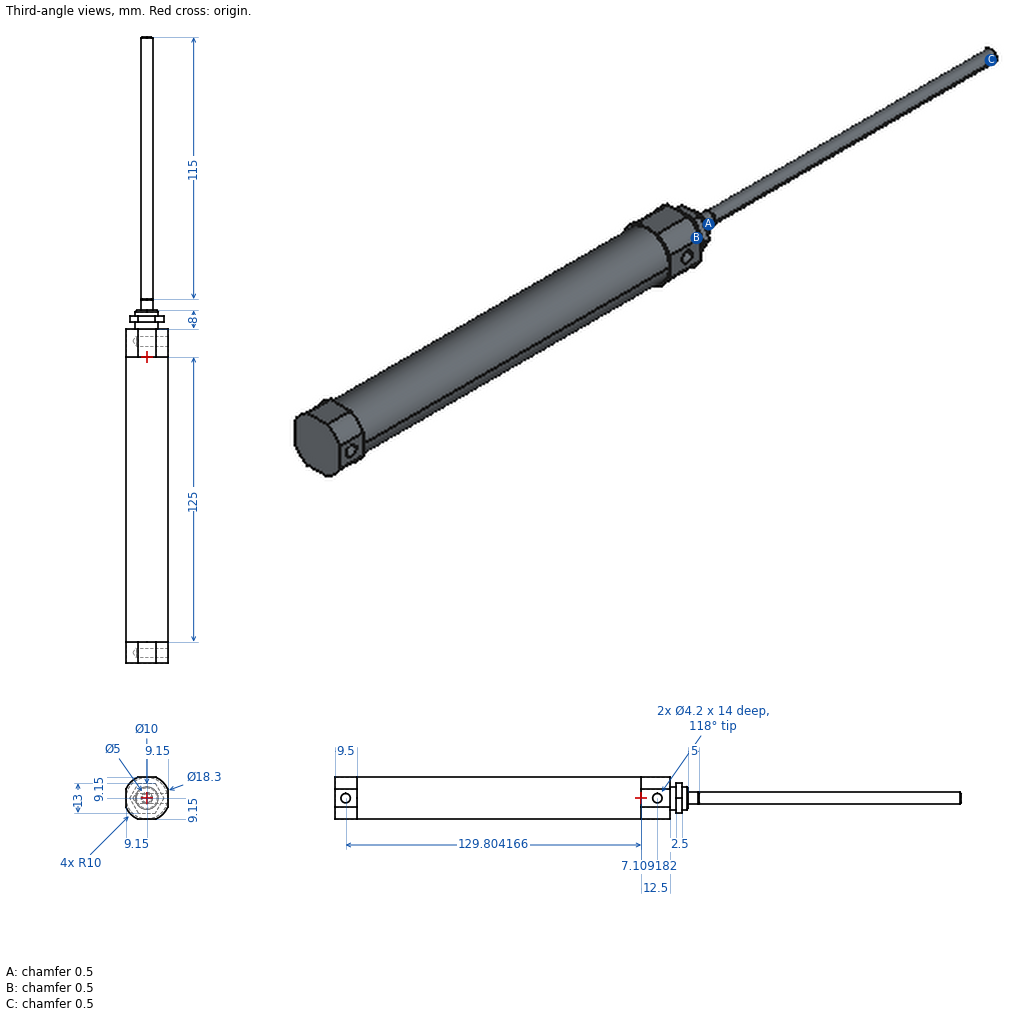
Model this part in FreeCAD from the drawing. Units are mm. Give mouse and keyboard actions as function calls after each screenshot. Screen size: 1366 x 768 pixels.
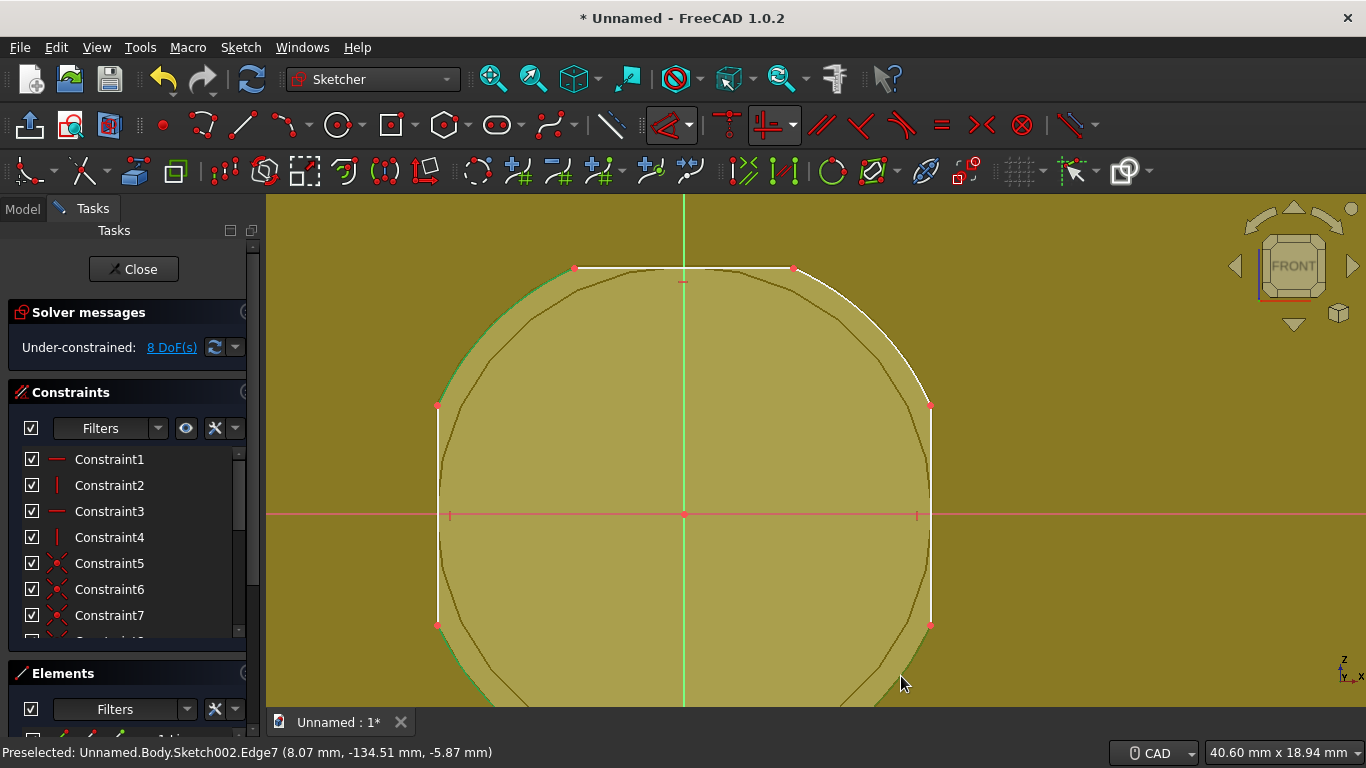
click(901, 354)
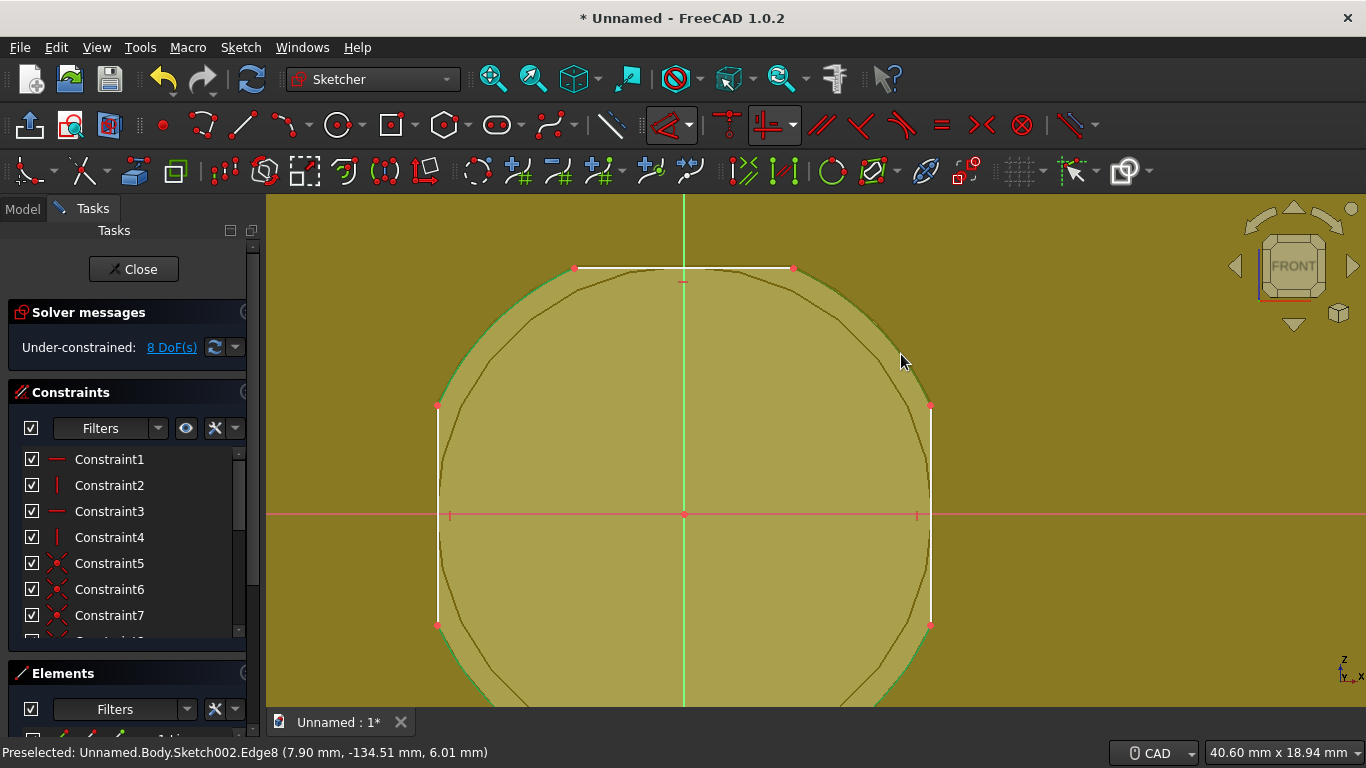
key(e)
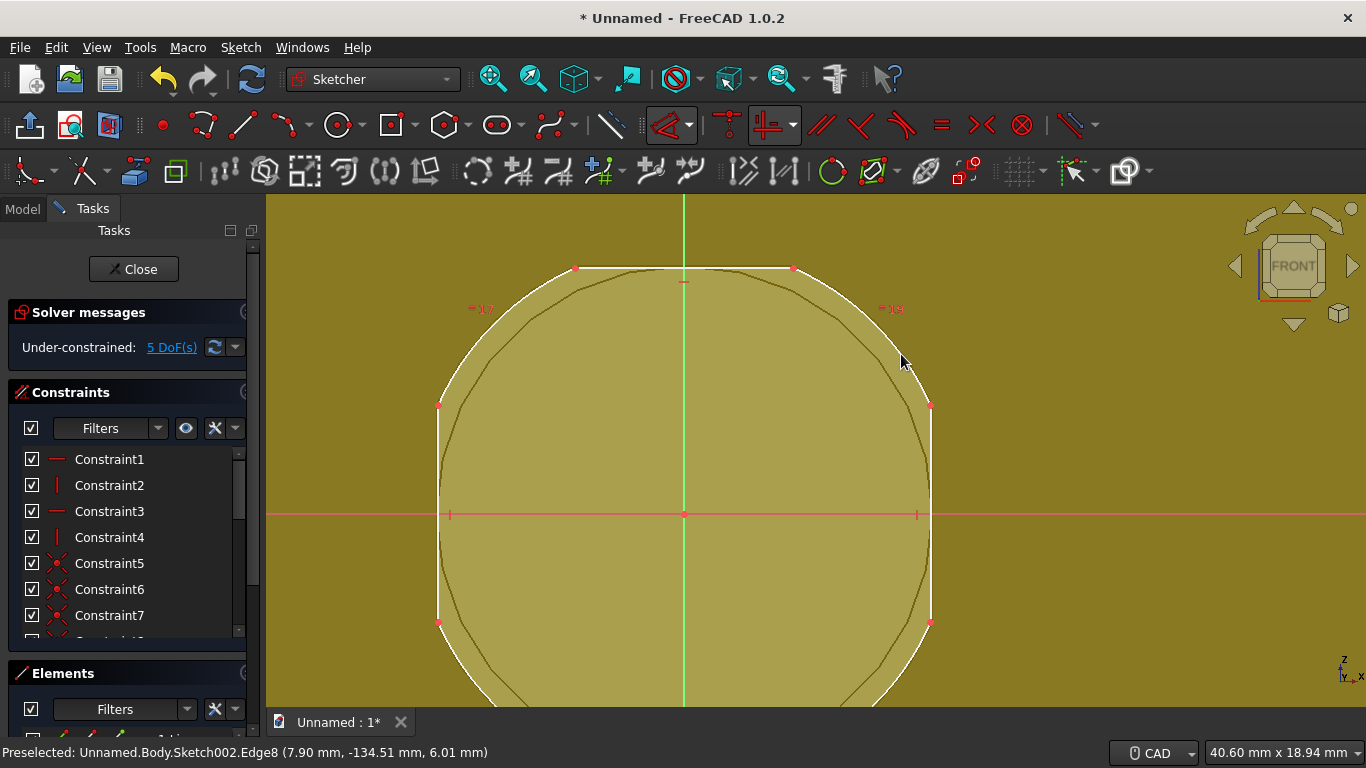
key(d)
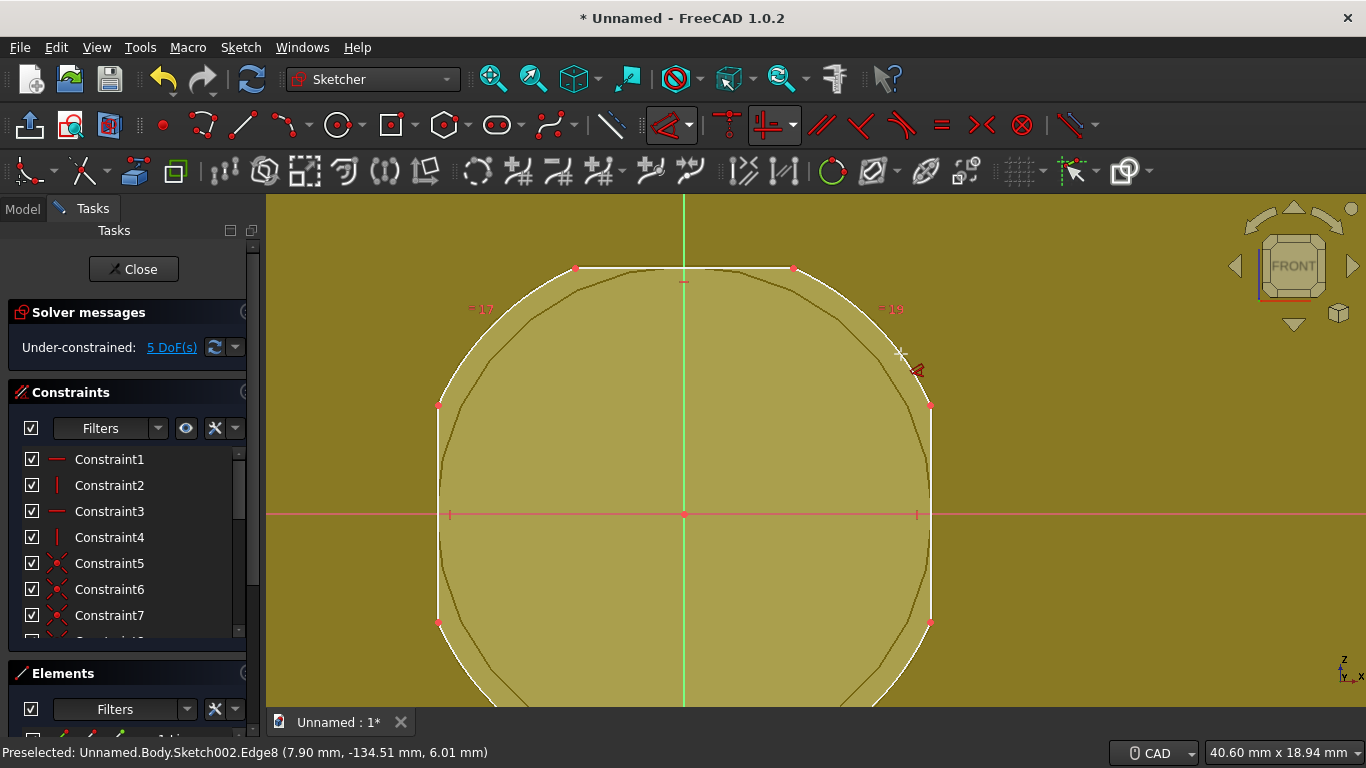
click(524, 298)
click(505, 272)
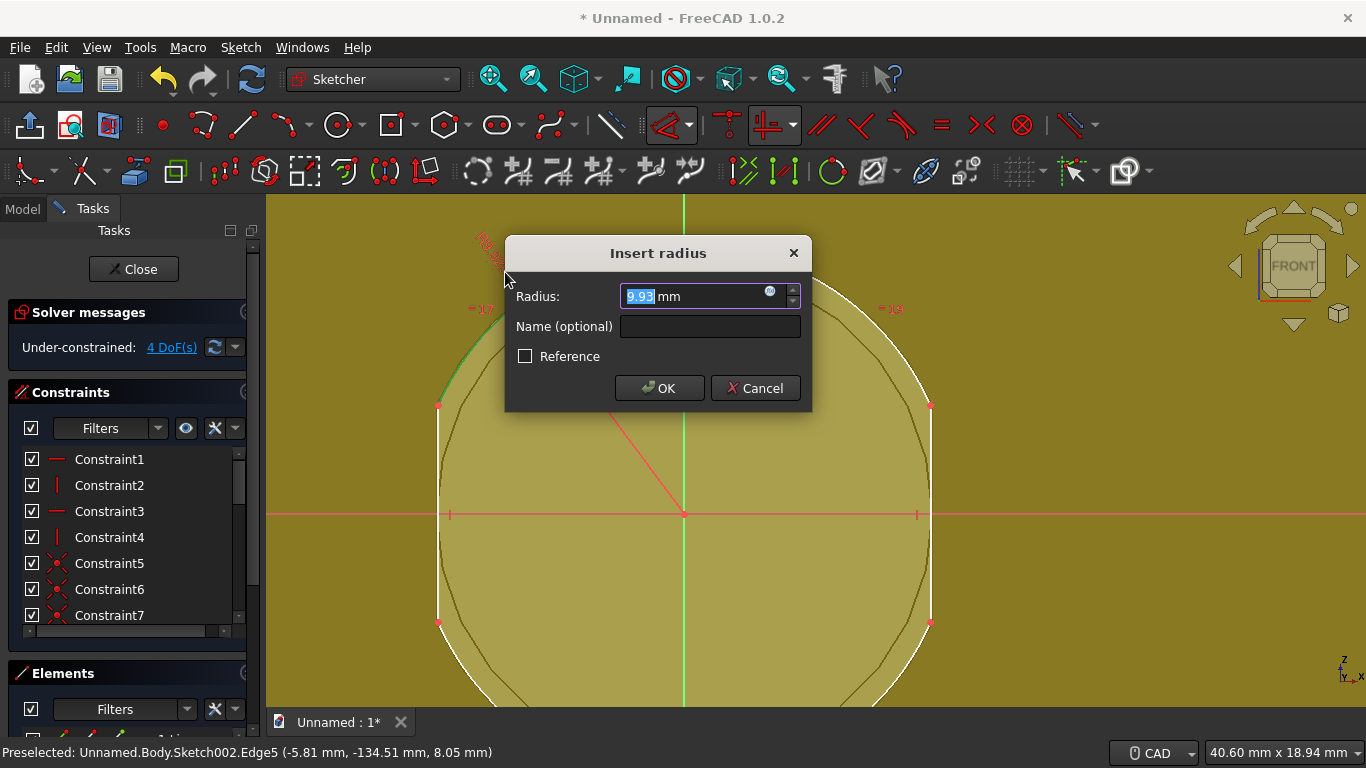
text(10)
key(Return)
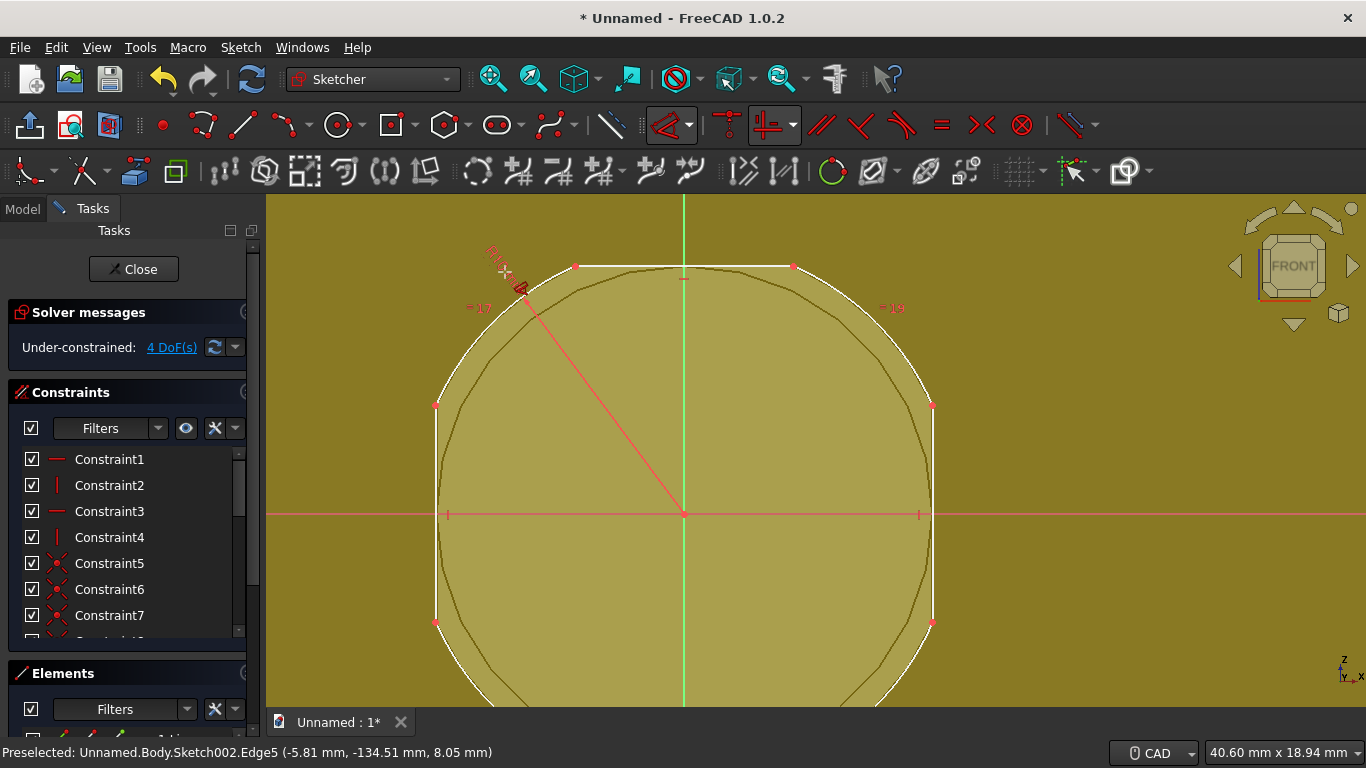
click(794, 266)
click(828, 390)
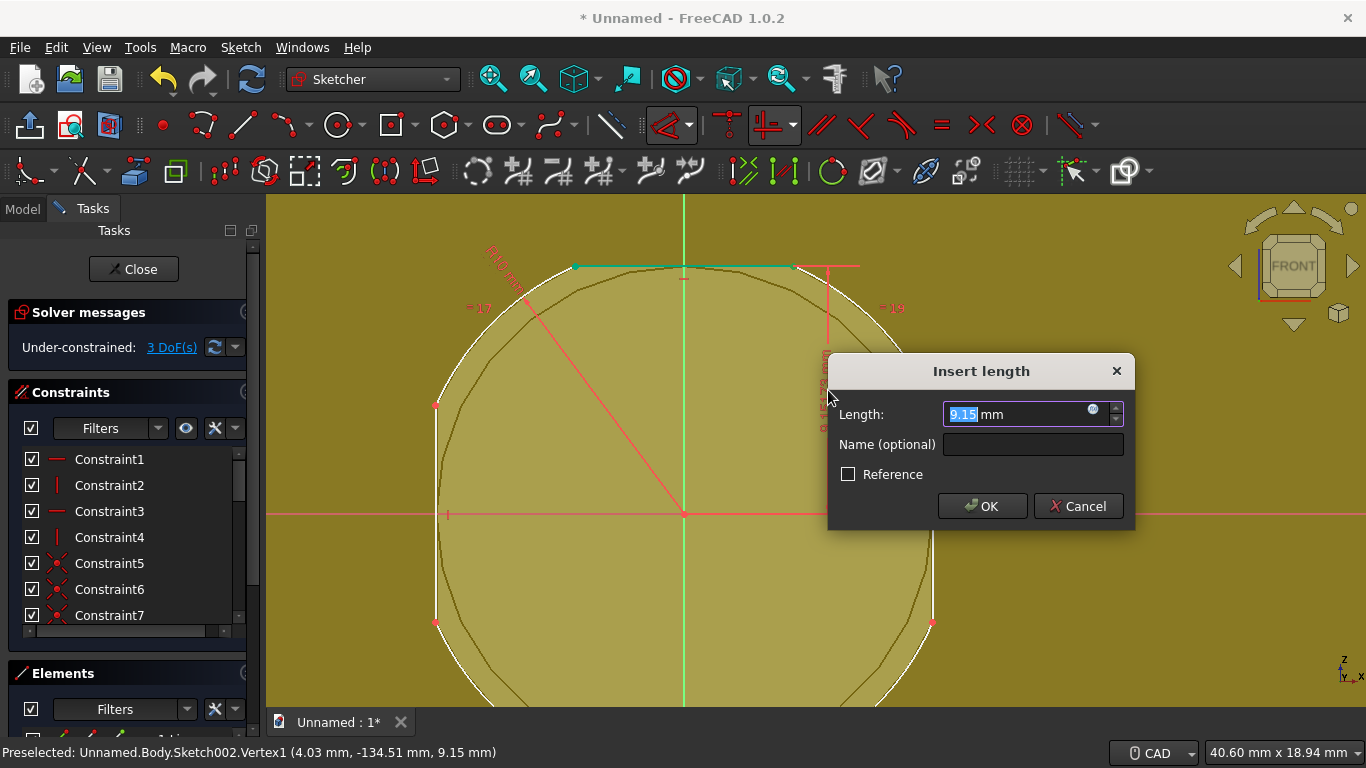
text(9.15)
key(Return)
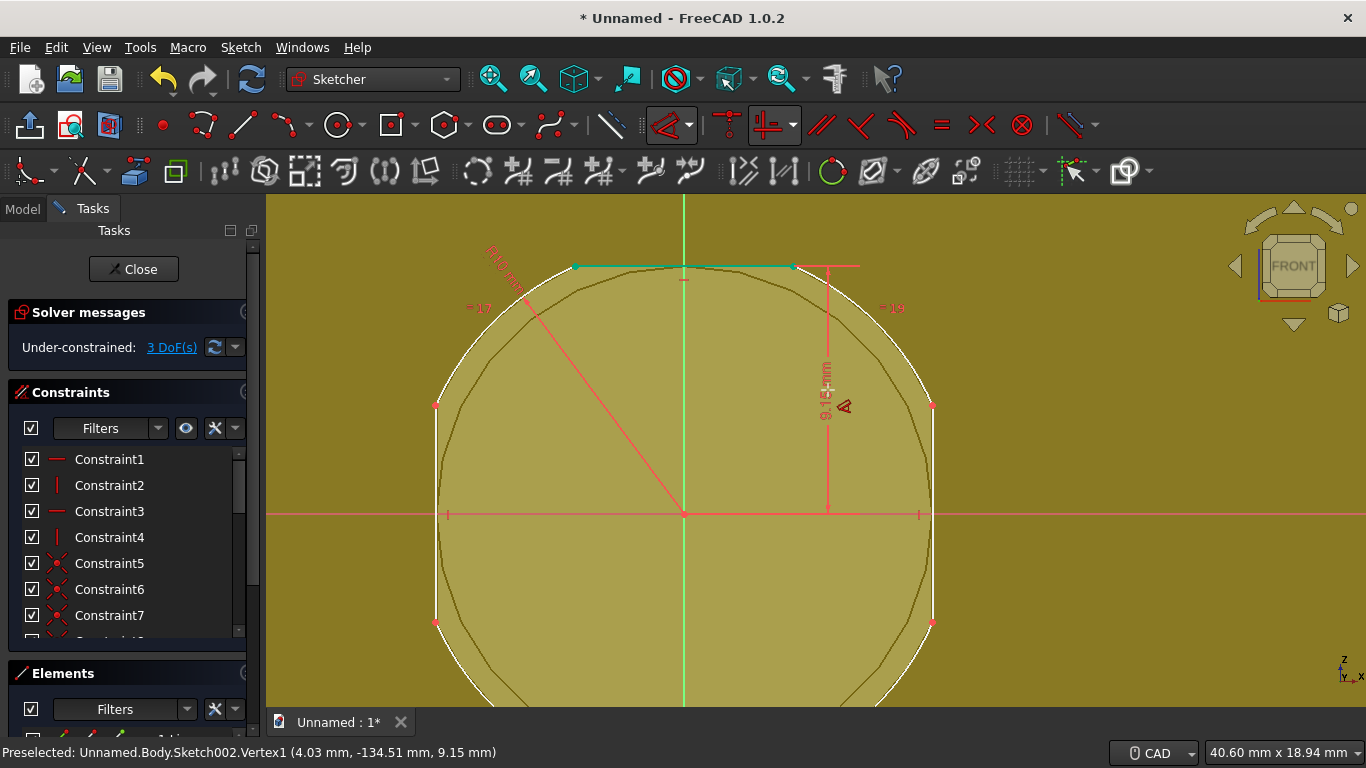
click(436, 406)
click(560, 372)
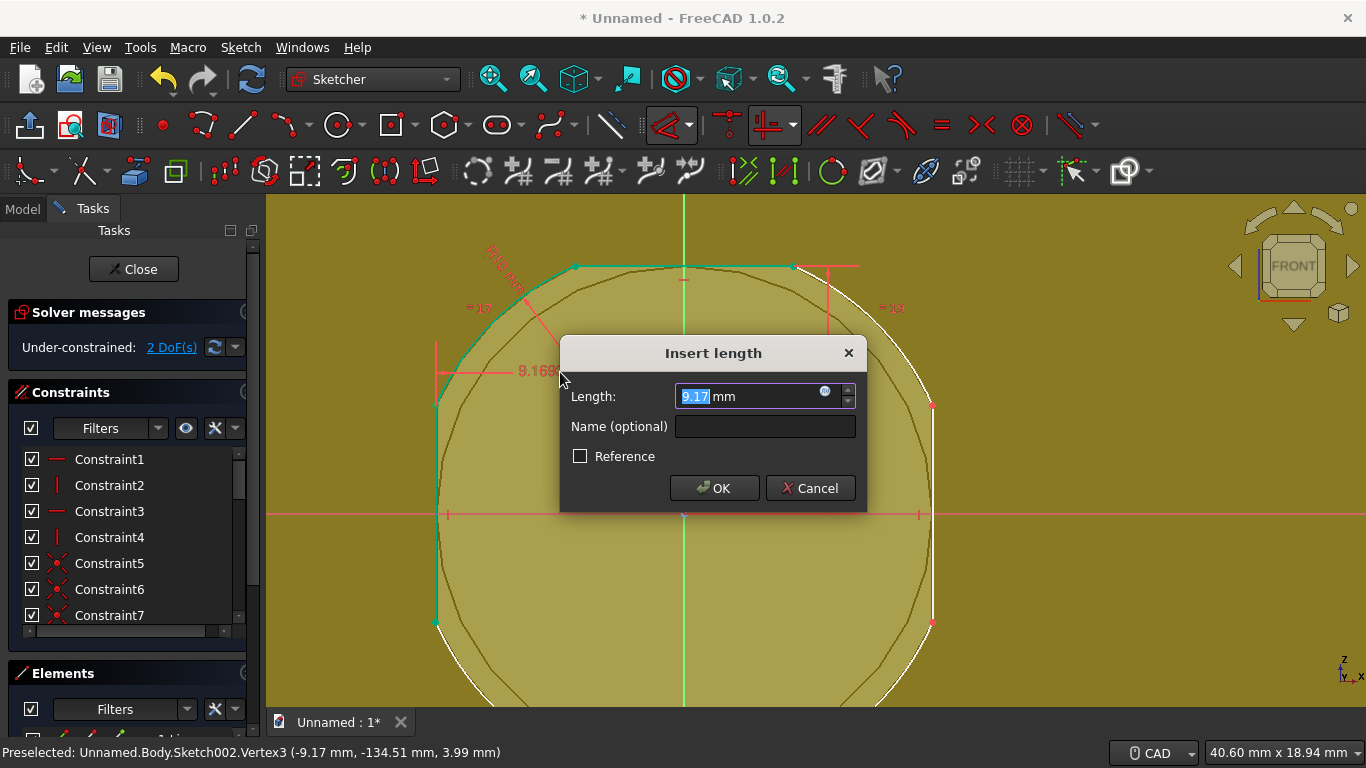
text(9.15)
key(Return)